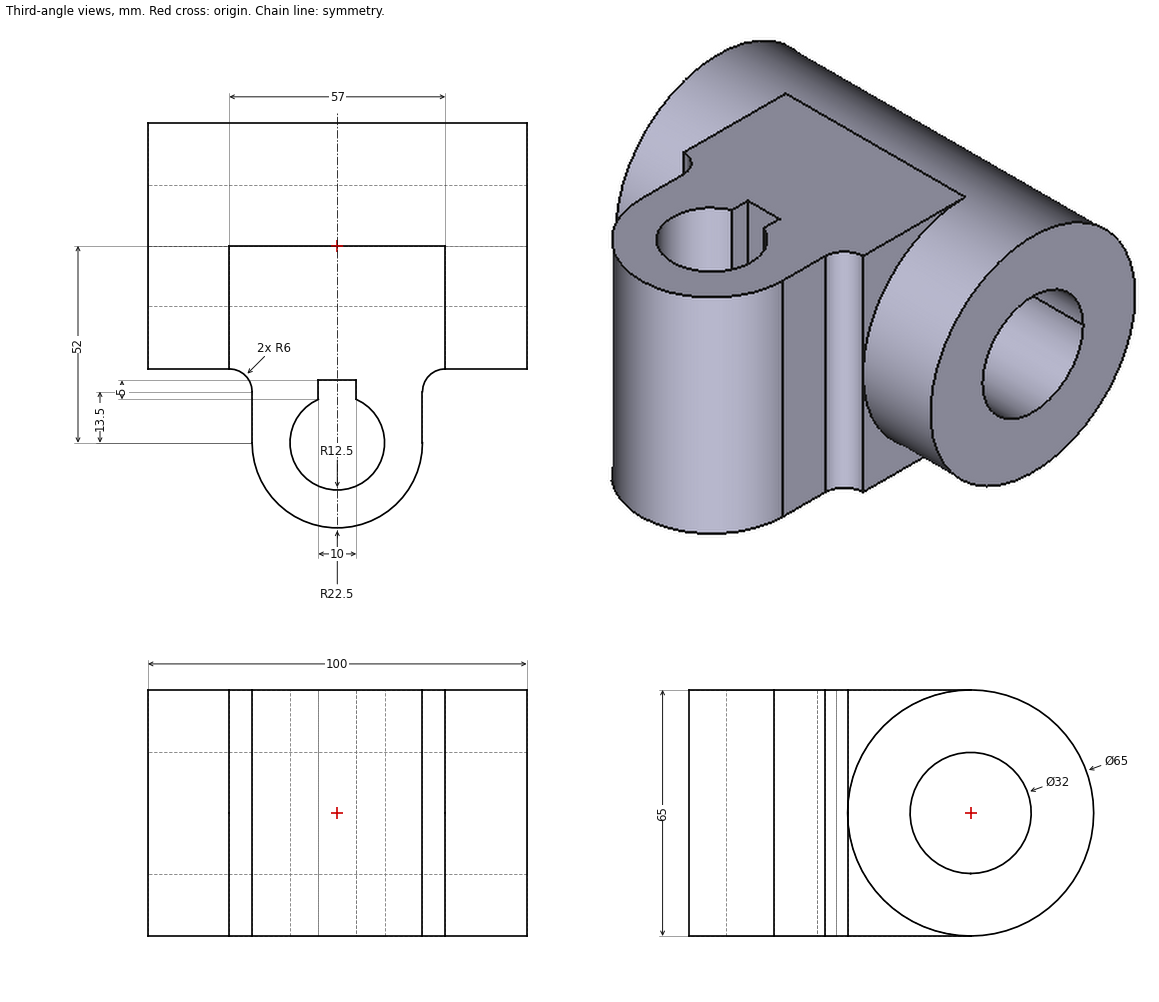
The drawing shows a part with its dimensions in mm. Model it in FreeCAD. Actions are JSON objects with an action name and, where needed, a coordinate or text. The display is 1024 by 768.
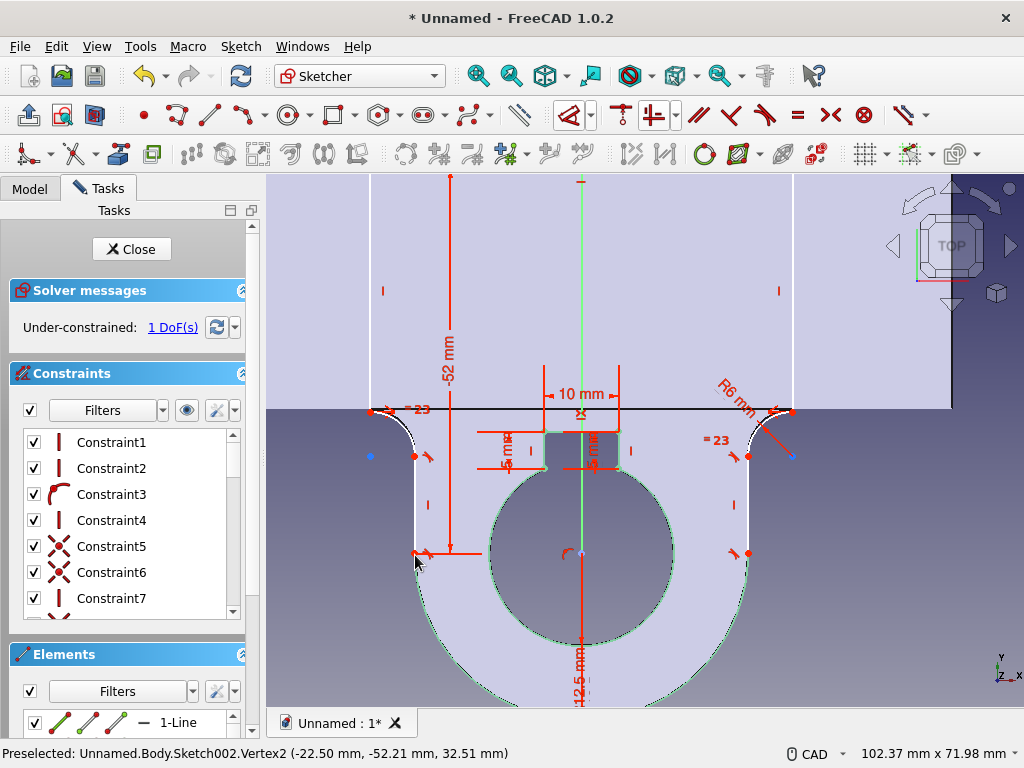
{"action": "left_click", "coordinate": [415, 486]}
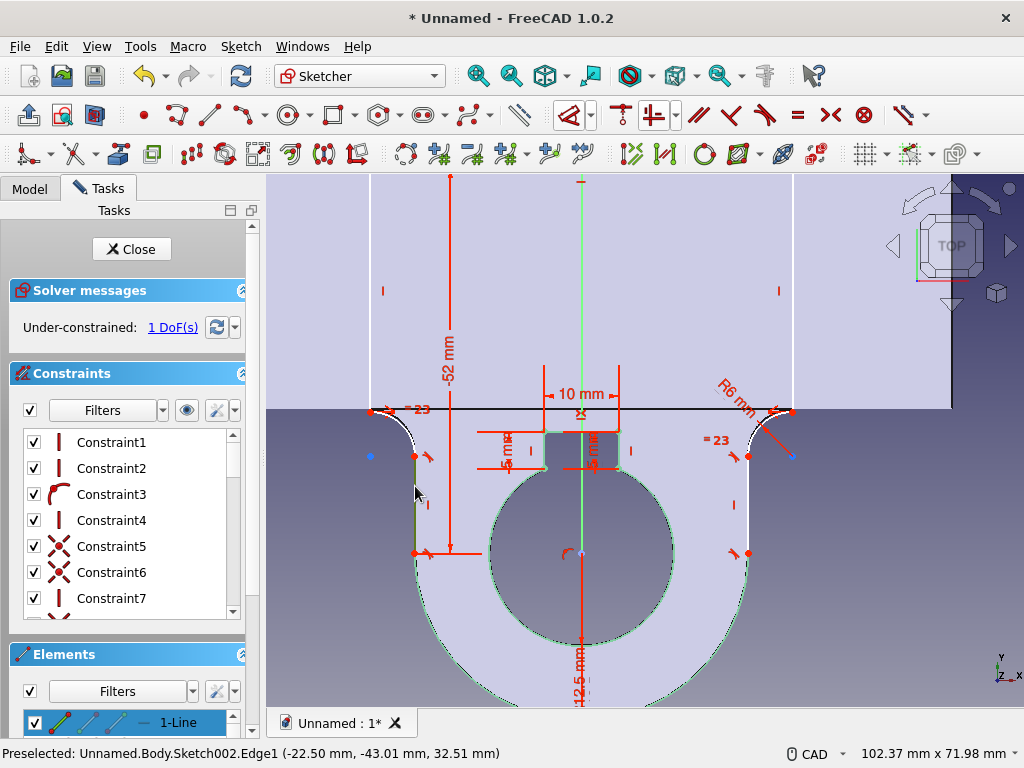
{"action": "key", "text": "i"}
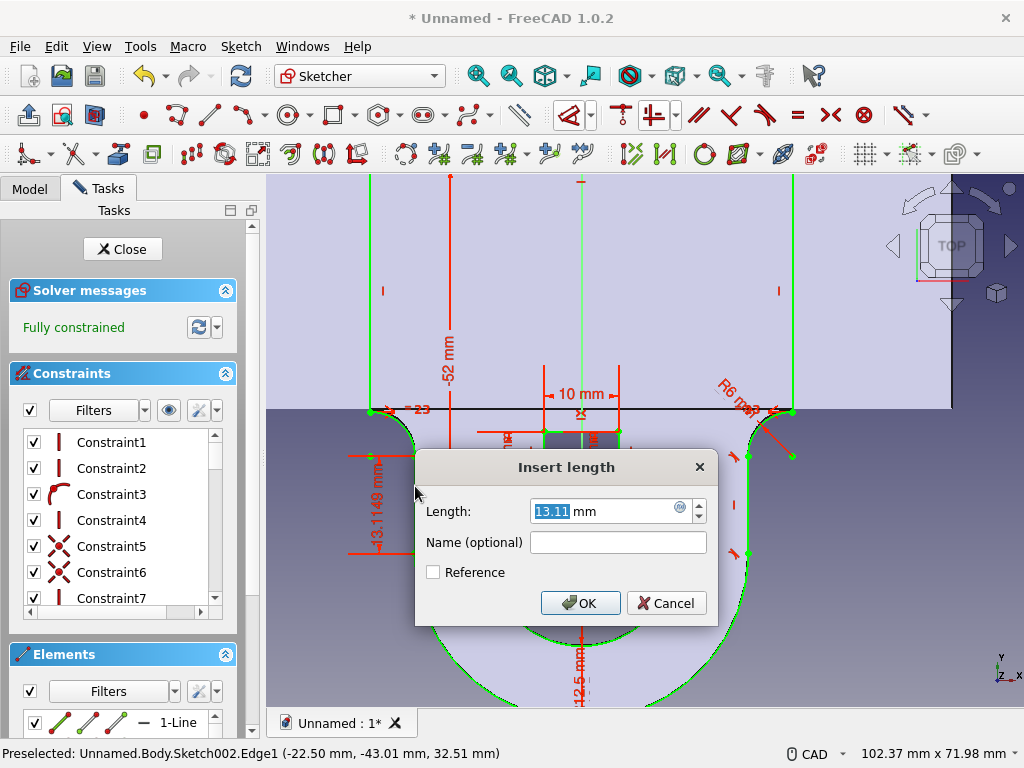
{"action": "type", "text": "13.5"}
{"action": "key", "text": "Return"}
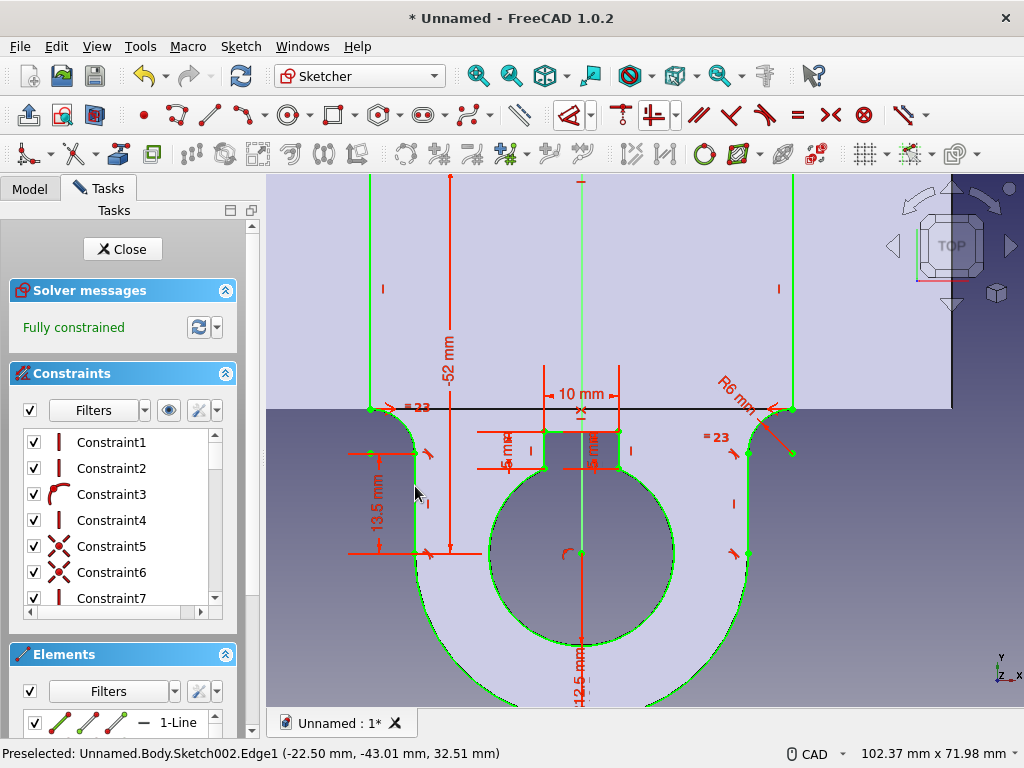
{"action": "left_click", "coordinate": [123, 249]}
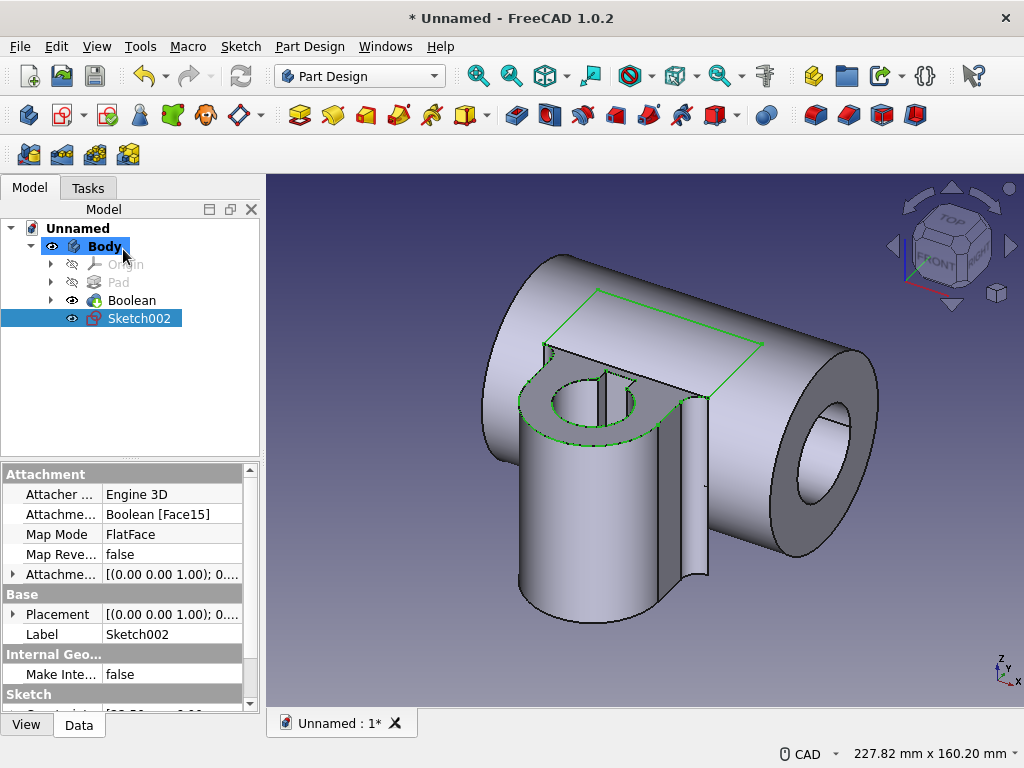
{"action": "left_click", "coordinate": [300, 116]}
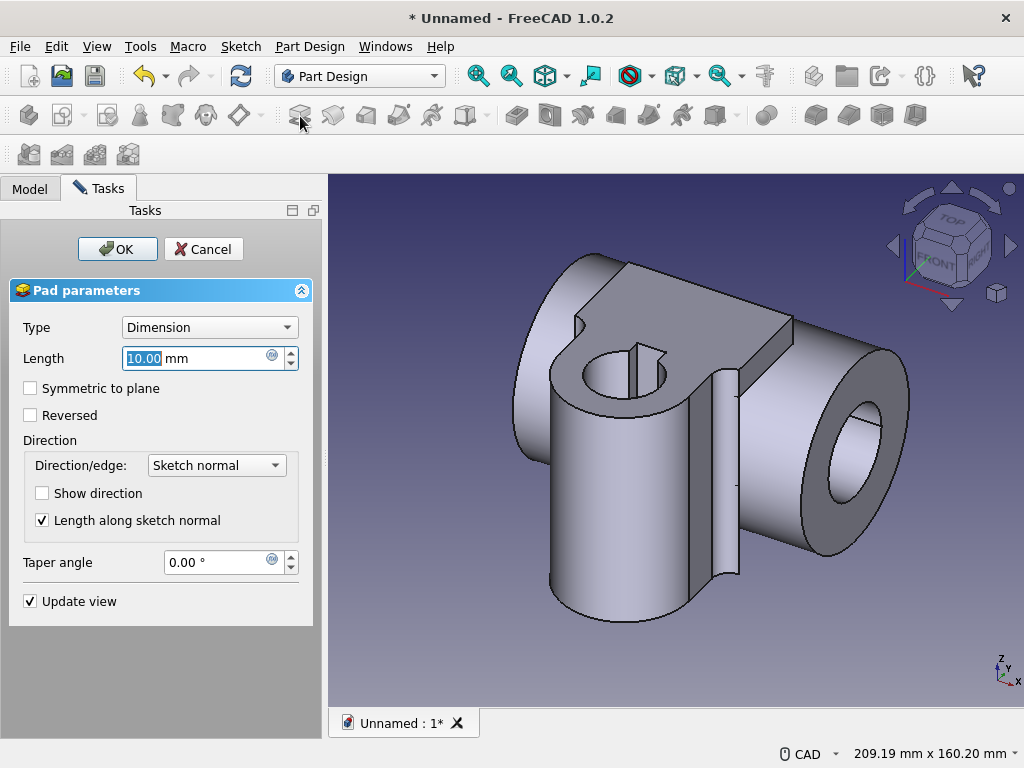
{"action": "type", "text": "65"}
{"action": "key", "text": "Tab"}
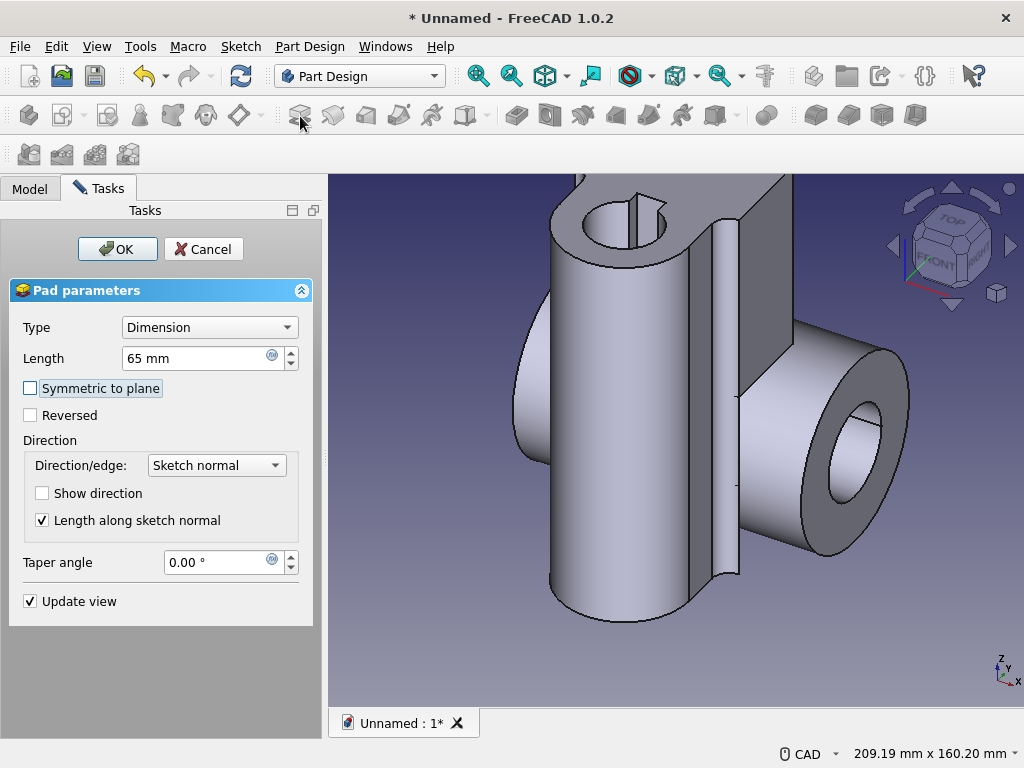
{"action": "left_click", "coordinate": [31, 415]}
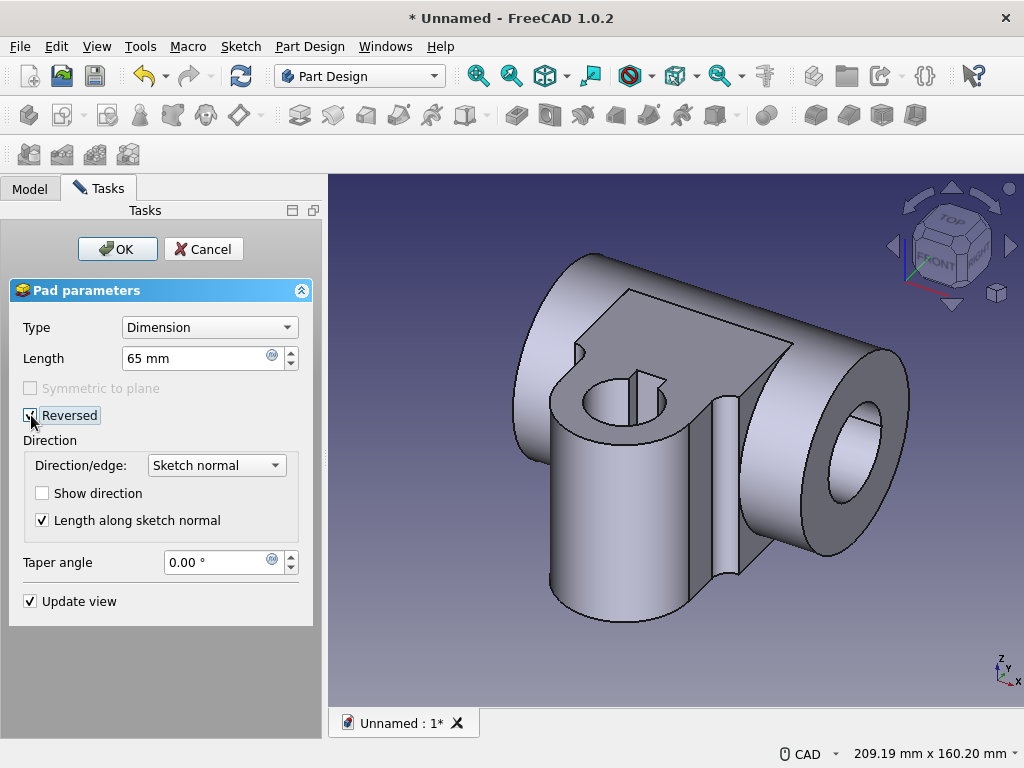
{"action": "left_click", "coordinate": [118, 249]}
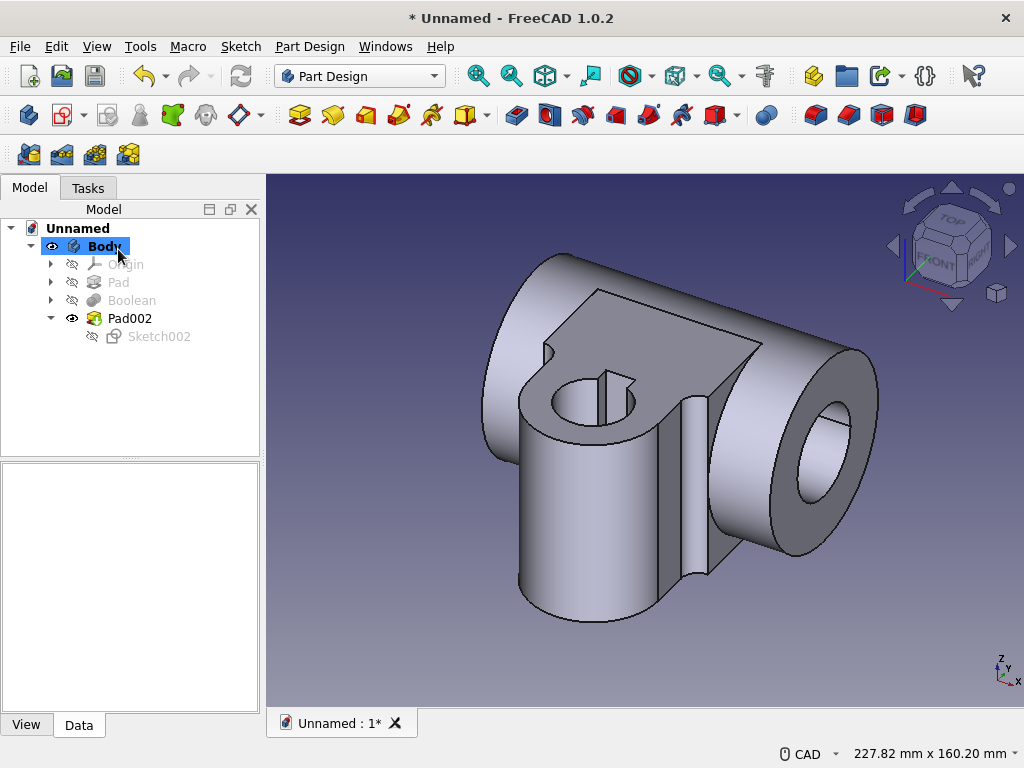
{"action": "left_click", "coordinate": [51, 264]}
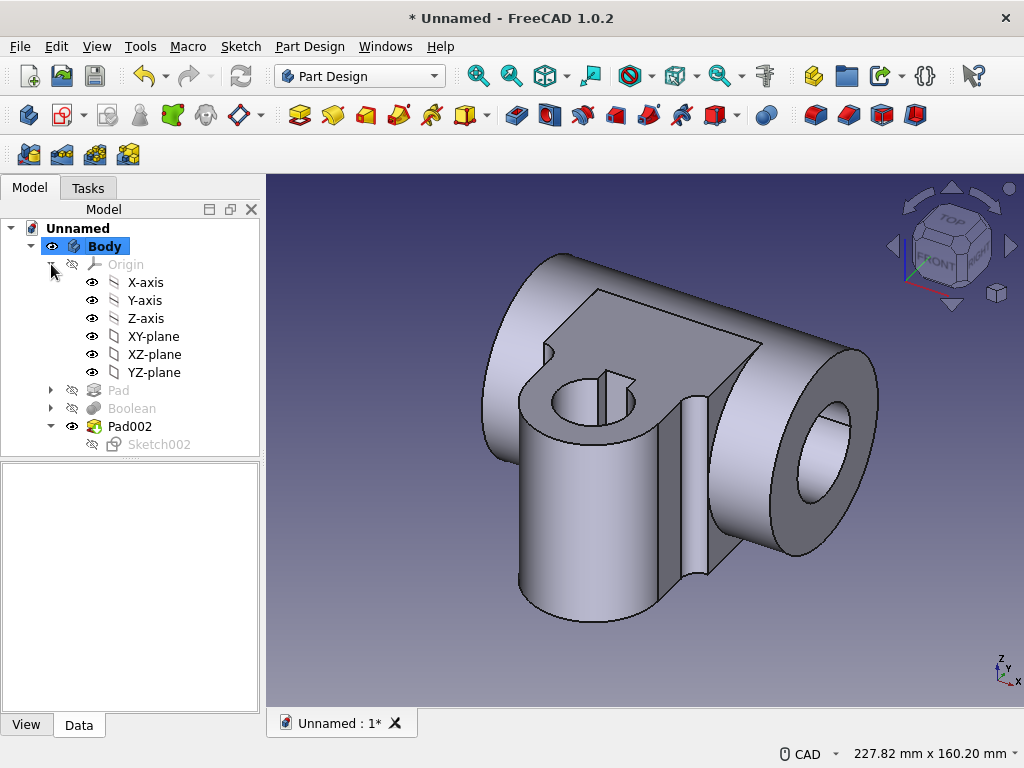
{"action": "left_click", "coordinate": [137, 372]}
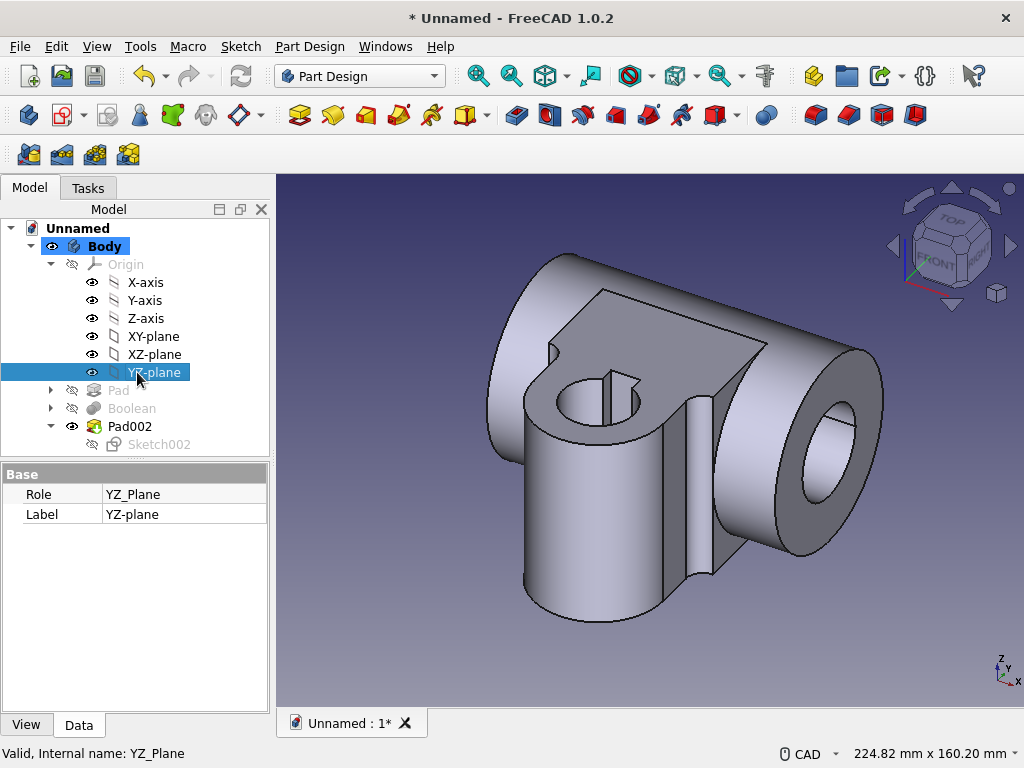
{"action": "left_click", "coordinate": [238, 116]}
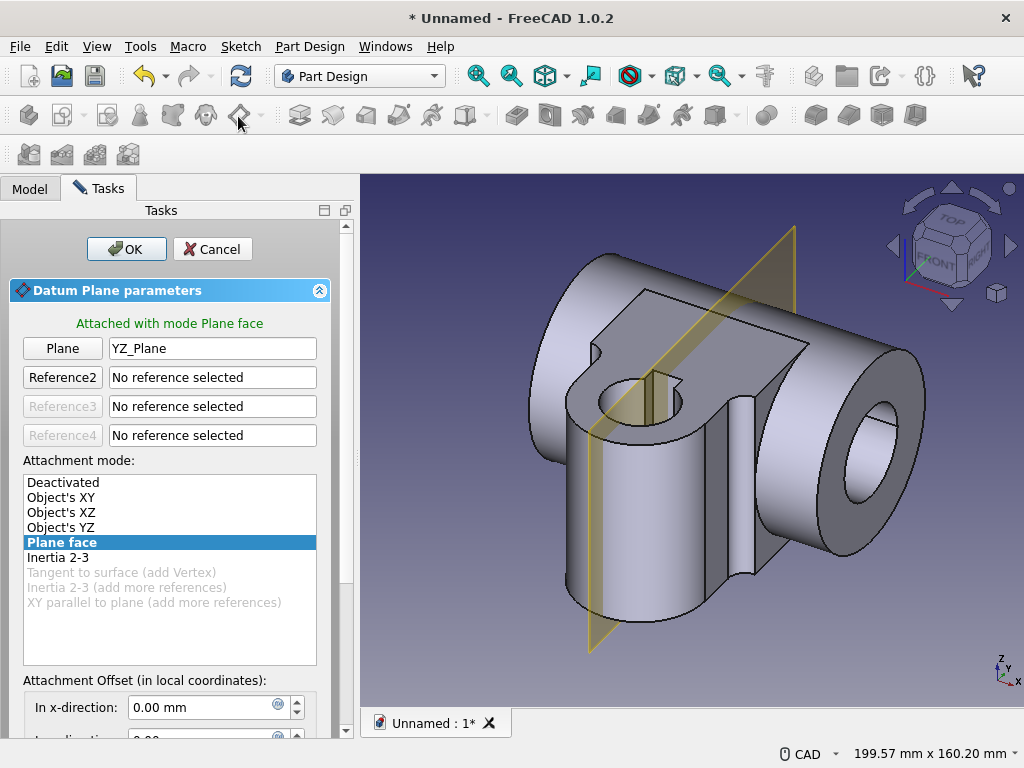
{"action": "scroll", "coordinate": [346, 479], "scroll_direction": "down", "scroll_amount": 2}